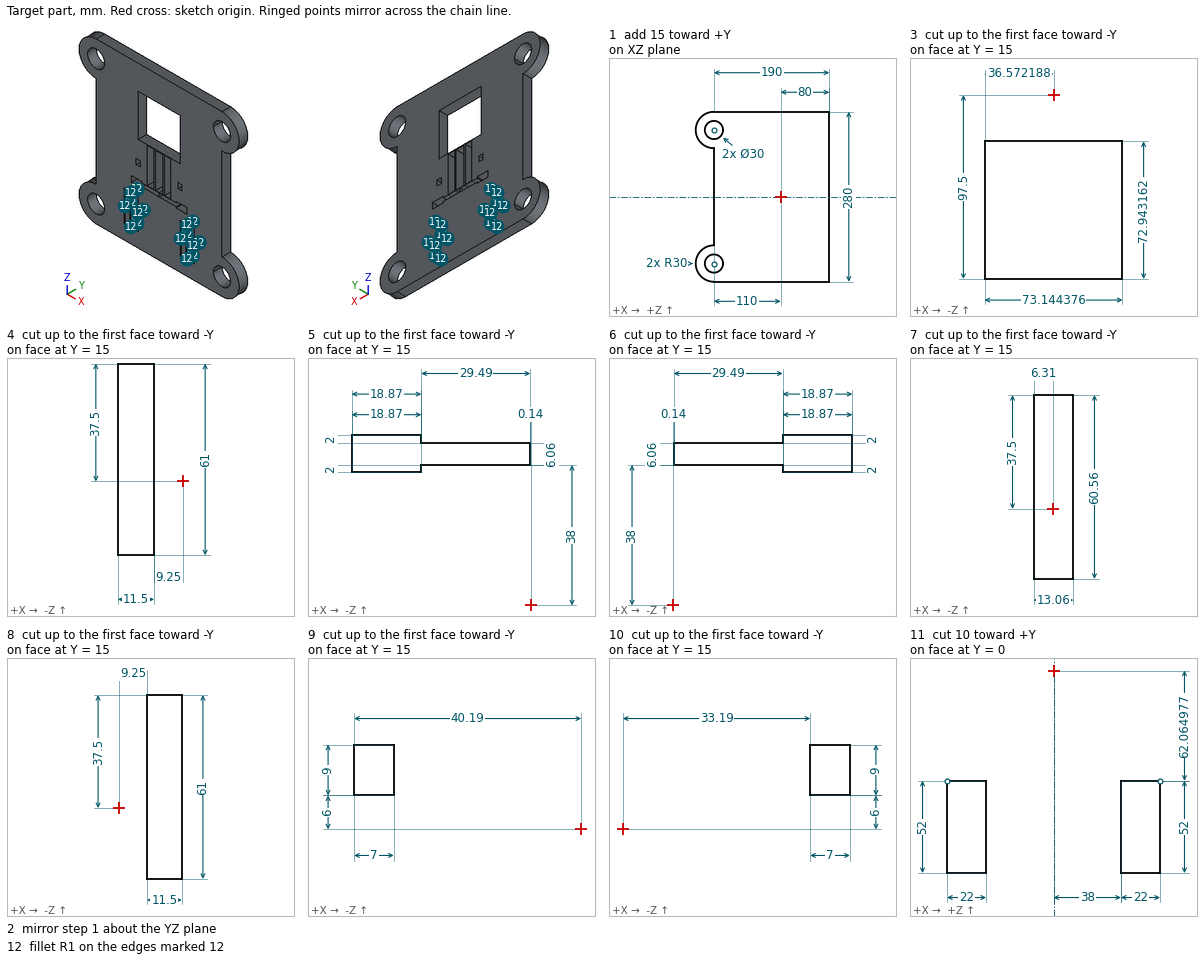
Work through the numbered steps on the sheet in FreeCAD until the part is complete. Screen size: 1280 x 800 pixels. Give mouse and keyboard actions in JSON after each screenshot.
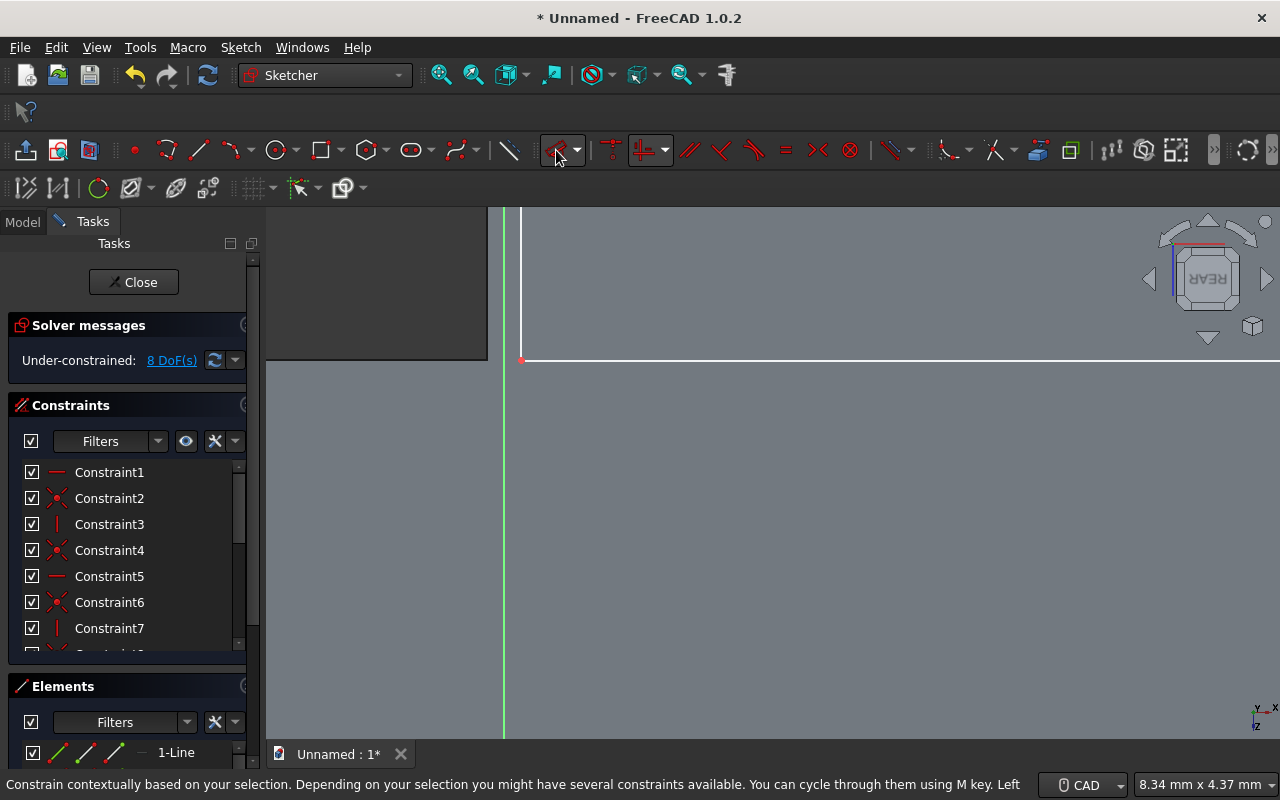
{"action": "scroll", "coordinate": [527, 362], "scroll_direction": "down", "scroll_amount": 14}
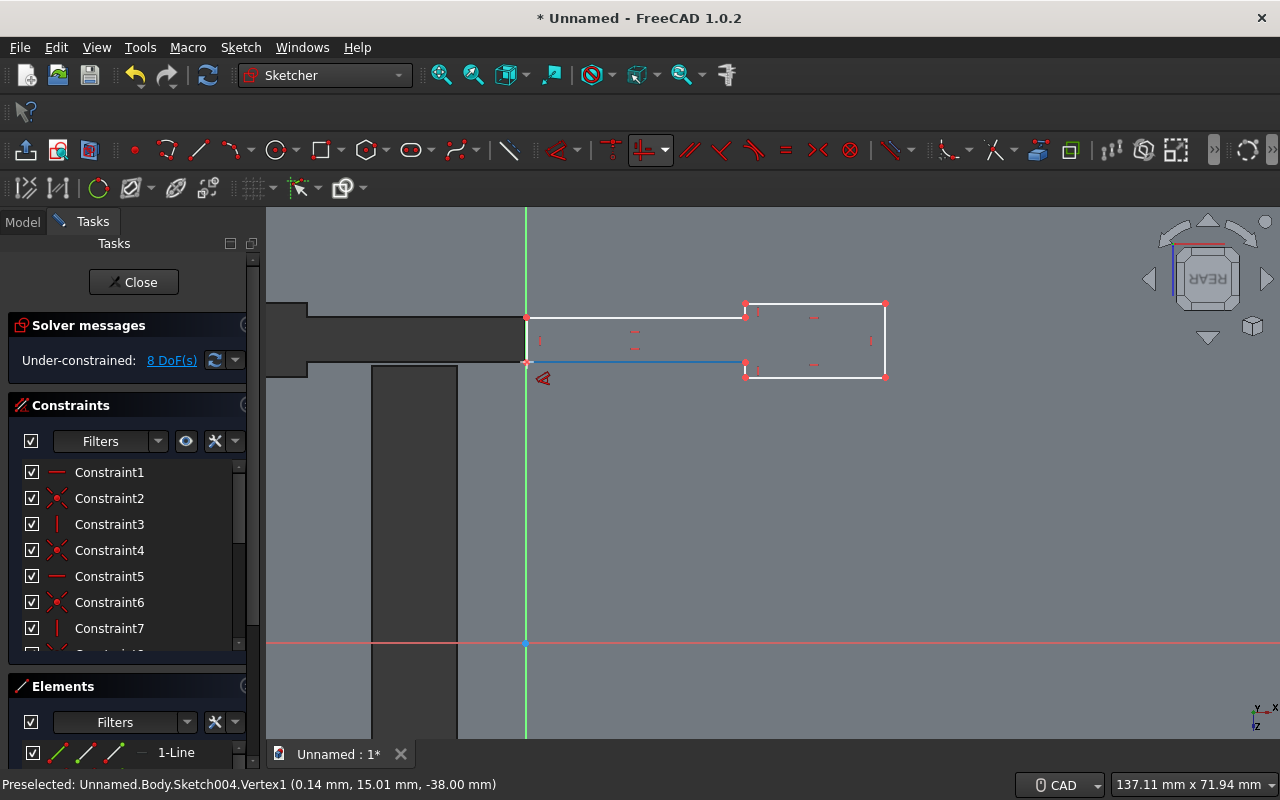
{"action": "scroll", "coordinate": [745, 367], "scroll_direction": "up", "scroll_amount": 6}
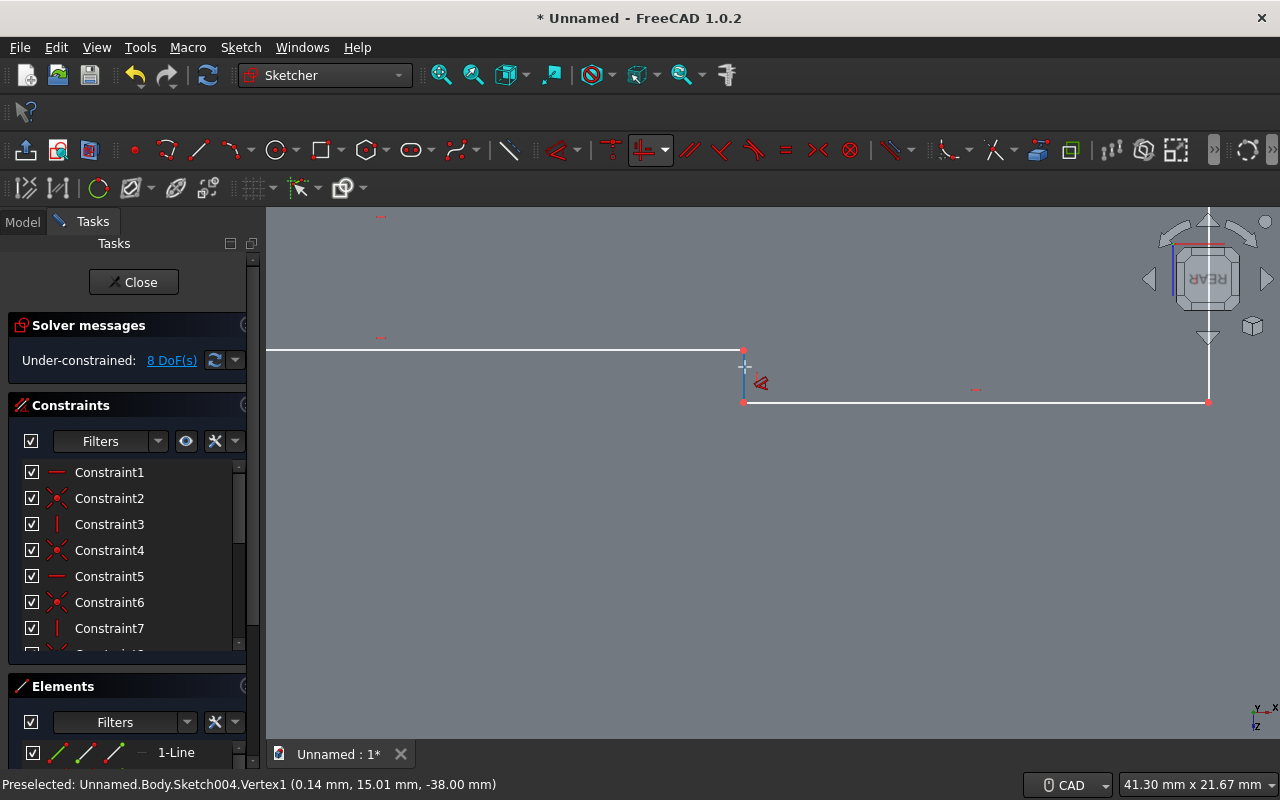
{"action": "left_click", "coordinate": [744, 366]}
{"action": "left_click", "coordinate": [778, 377]}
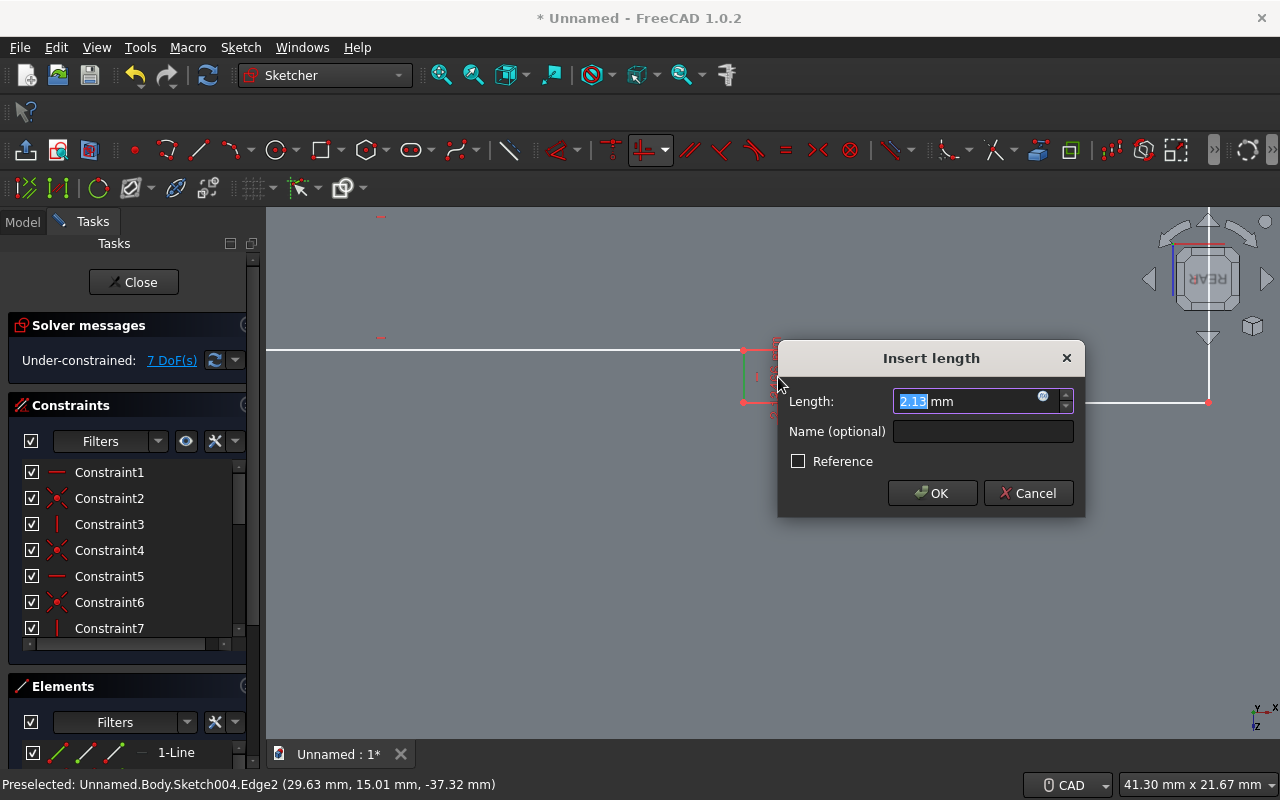
{"action": "type", "text": "2"}
{"action": "key", "text": "Return"}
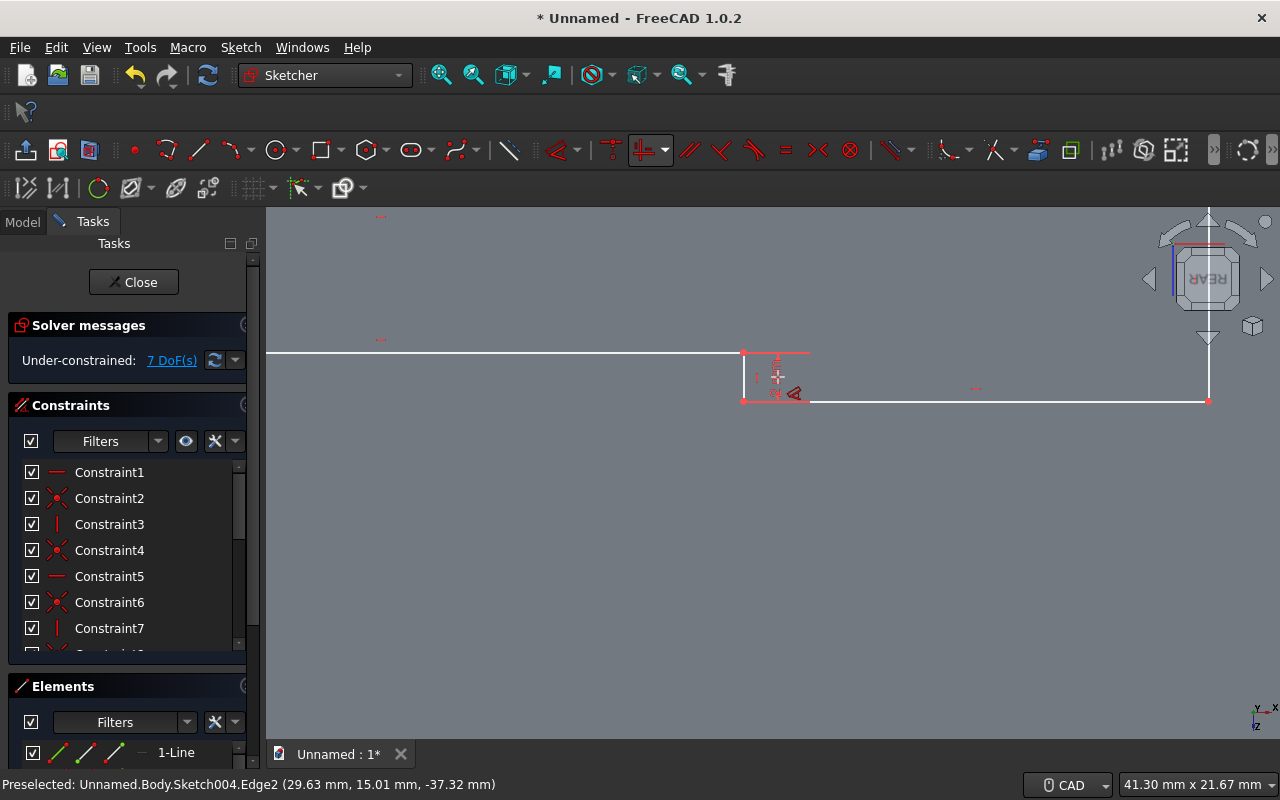
{"action": "scroll", "coordinate": [744, 367], "scroll_direction": "down", "scroll_amount": 6}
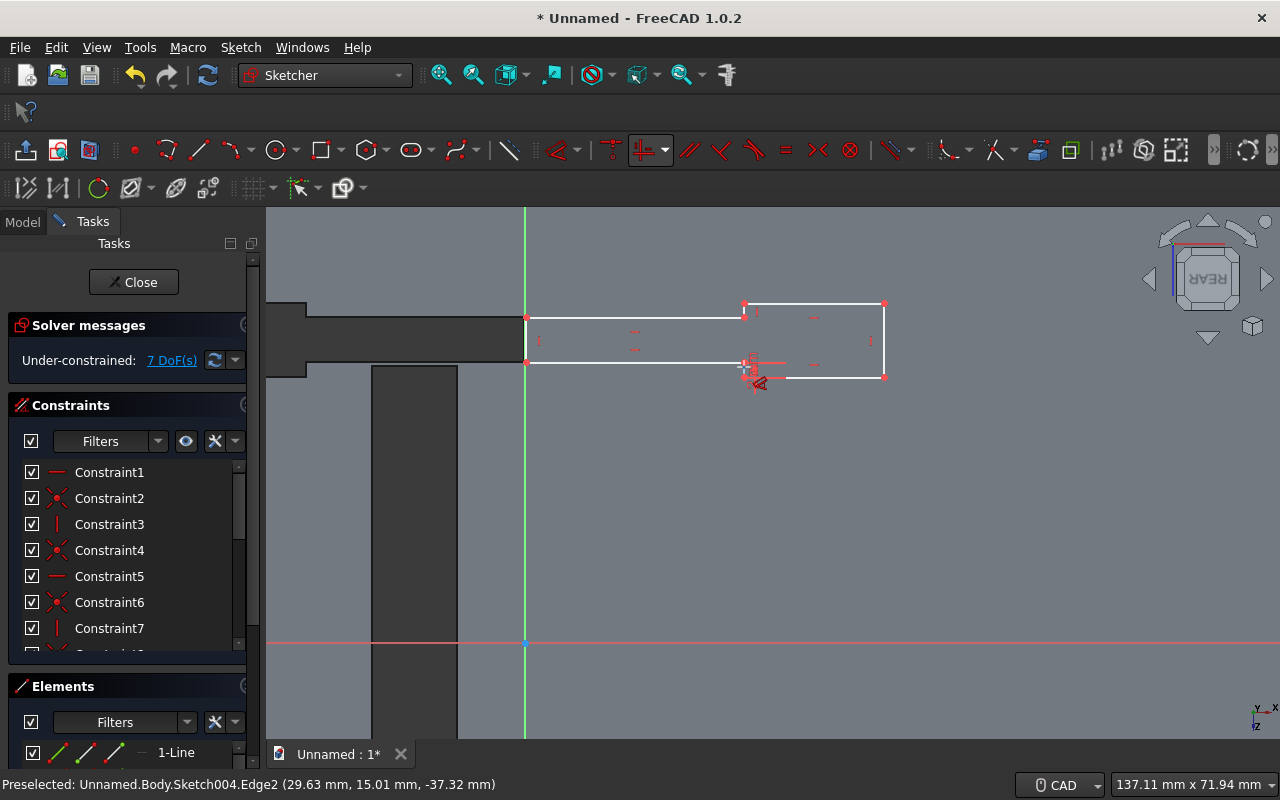
{"action": "scroll", "coordinate": [744, 308], "scroll_direction": "up", "scroll_amount": 6}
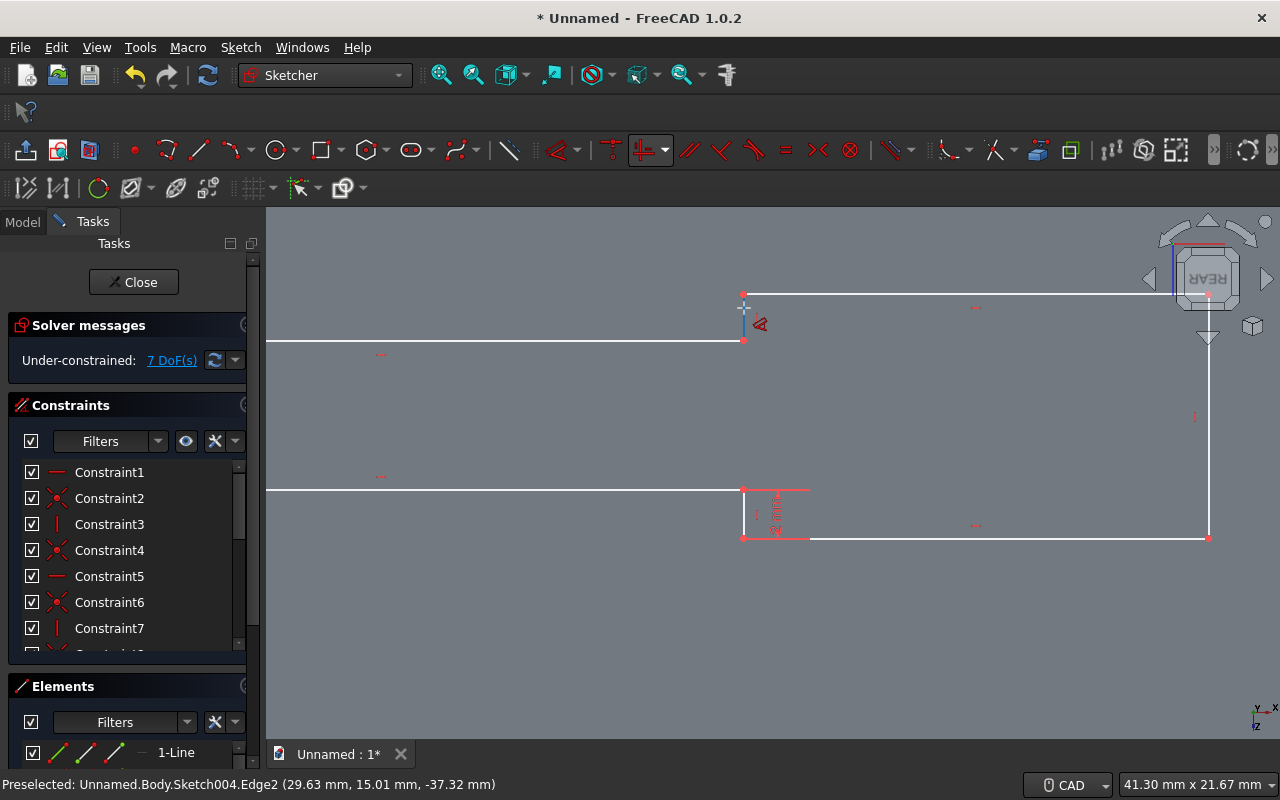
{"action": "left_click", "coordinate": [744, 308]}
{"action": "left_click", "coordinate": [778, 318]}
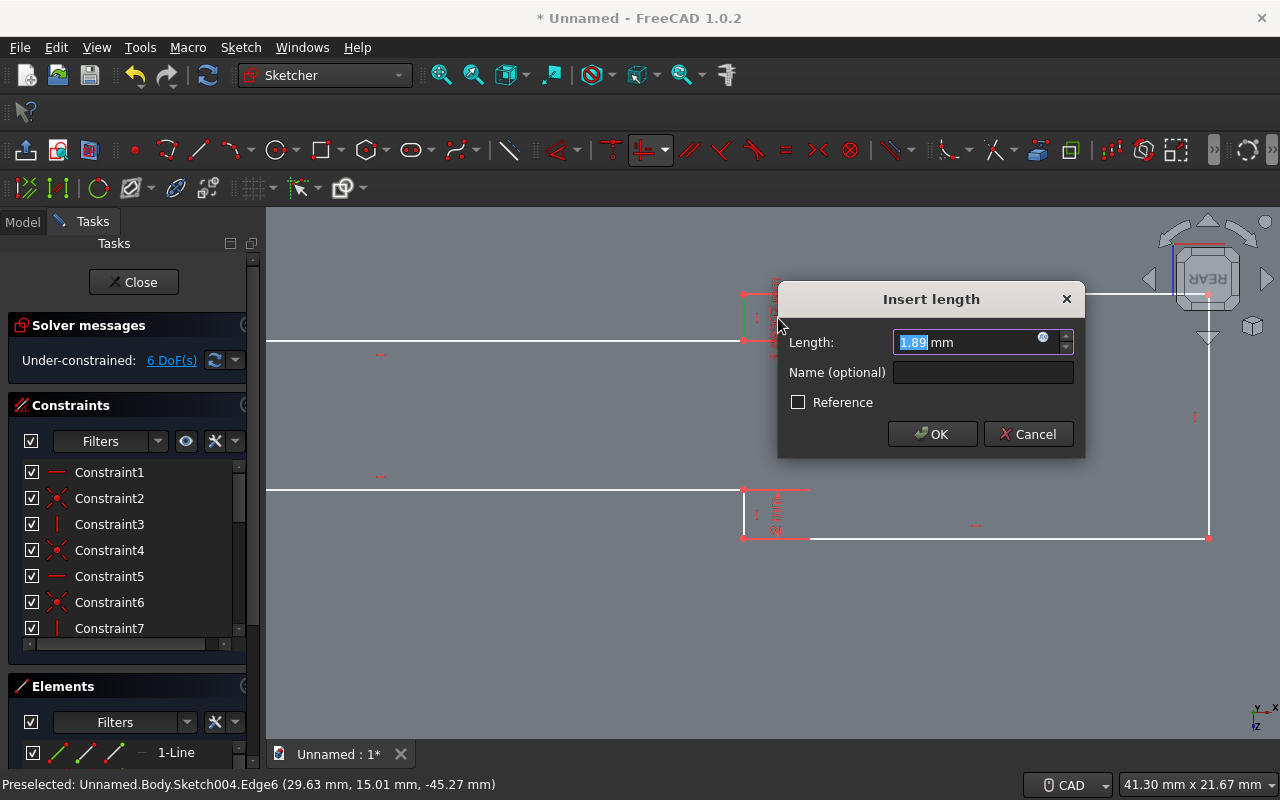
{"action": "type", "text": "2"}
{"action": "key", "text": "Return"}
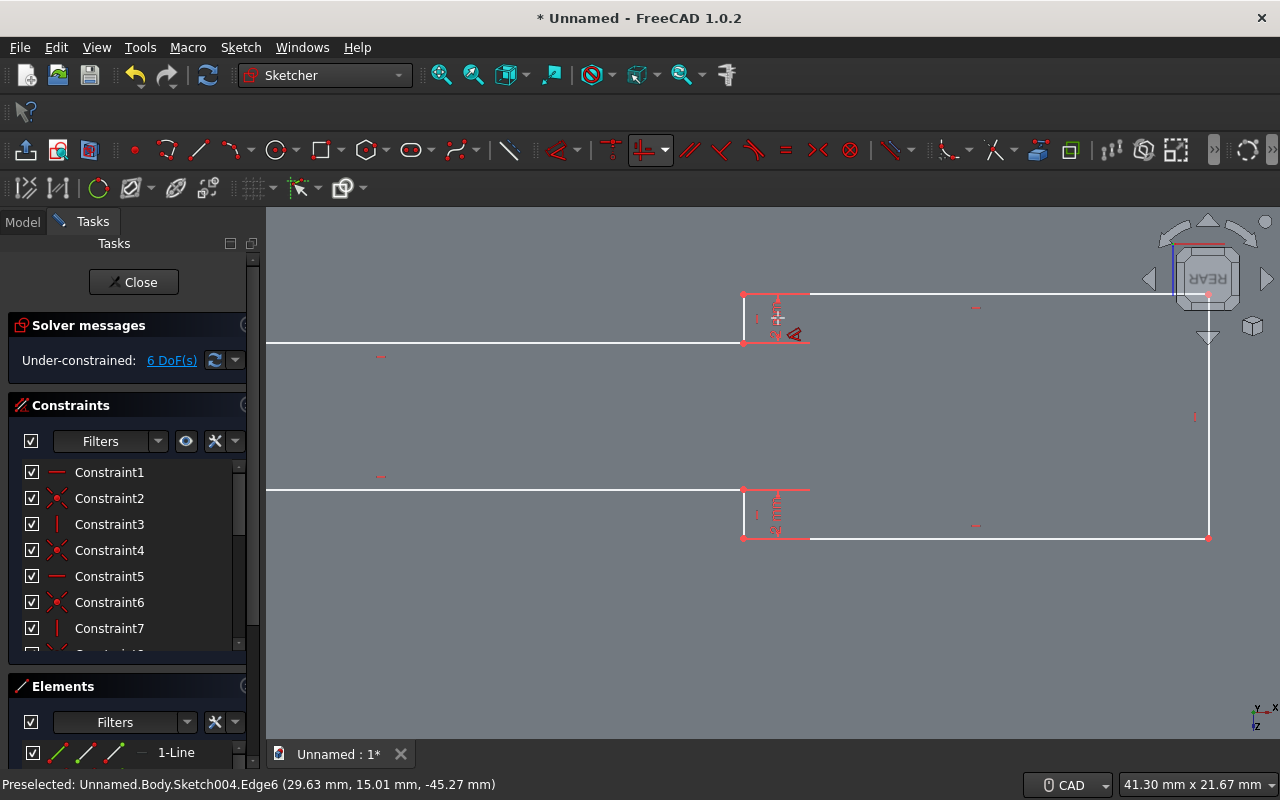
{"action": "scroll", "coordinate": [744, 308], "scroll_direction": "down", "scroll_amount": 6}